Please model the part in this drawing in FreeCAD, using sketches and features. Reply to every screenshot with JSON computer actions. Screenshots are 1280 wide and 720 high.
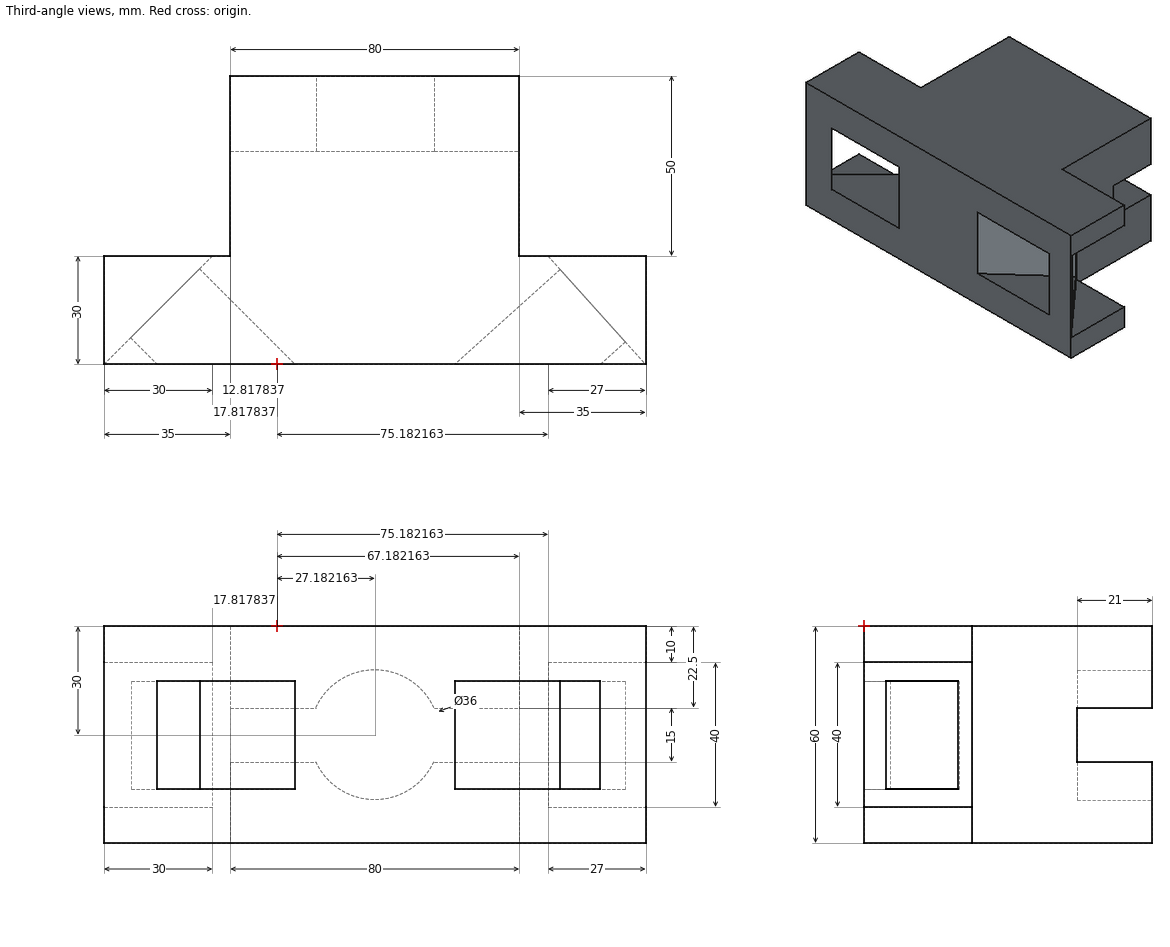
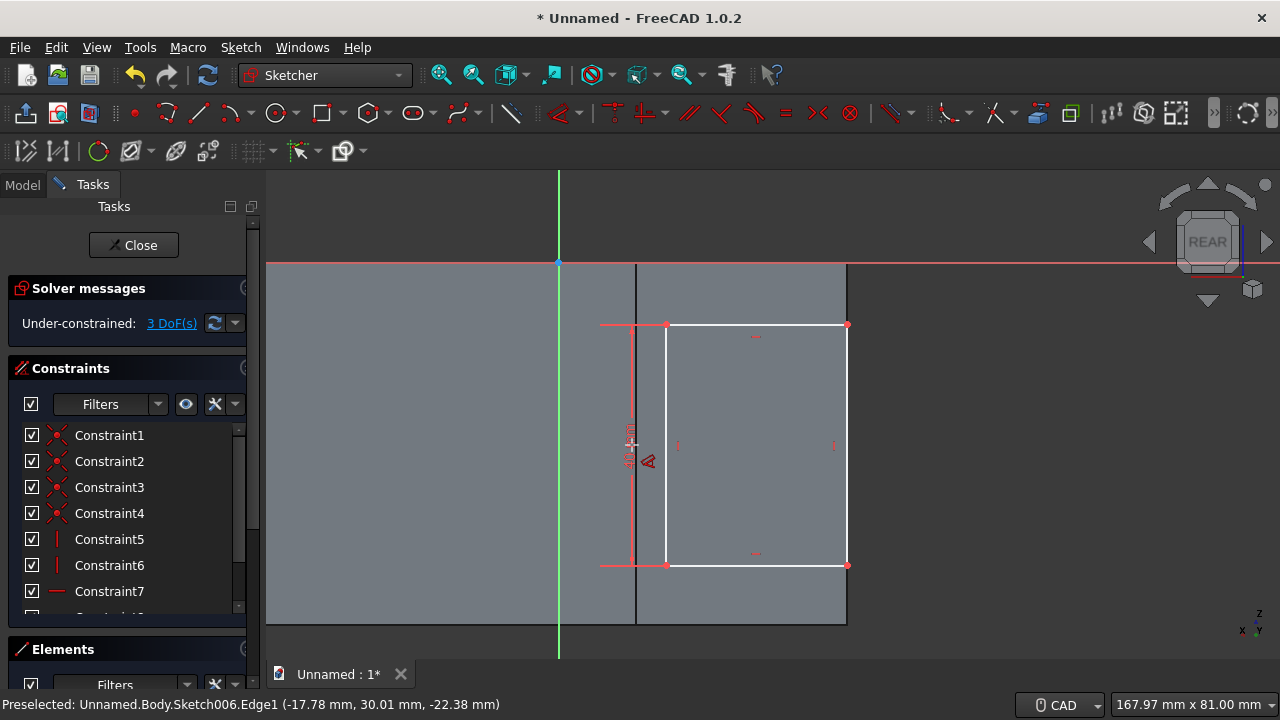
{"action": "left_click", "coordinate": [720, 566]}
{"action": "left_click", "coordinate": [757, 600]}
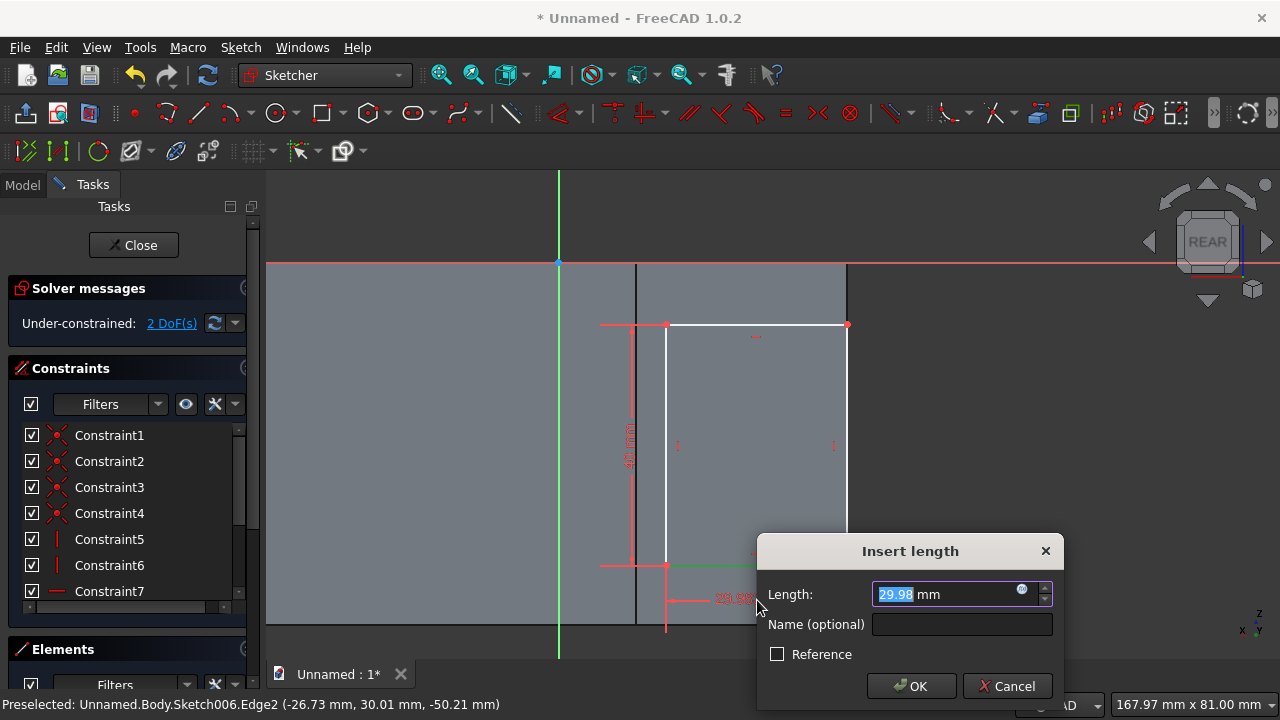
{"action": "type", "text": "30"}
{"action": "key", "text": "Return"}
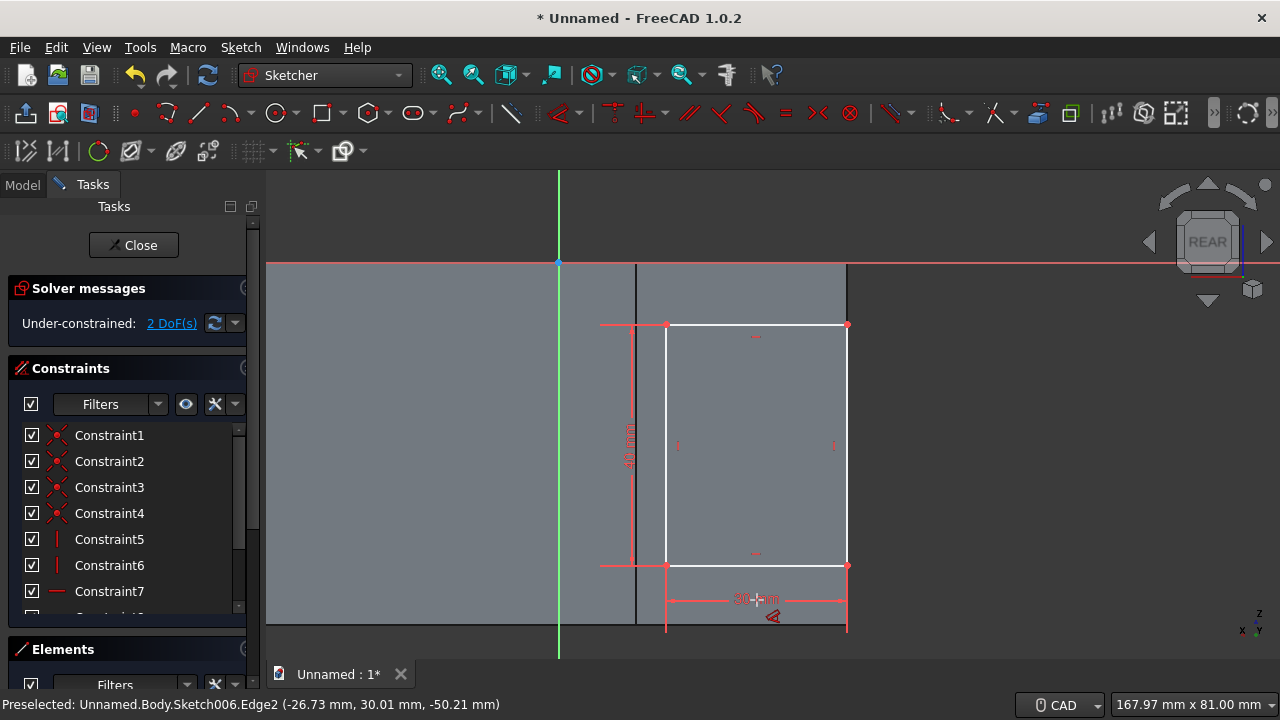
{"action": "left_click", "coordinate": [666, 325]}
{"action": "left_click", "coordinate": [525, 294]}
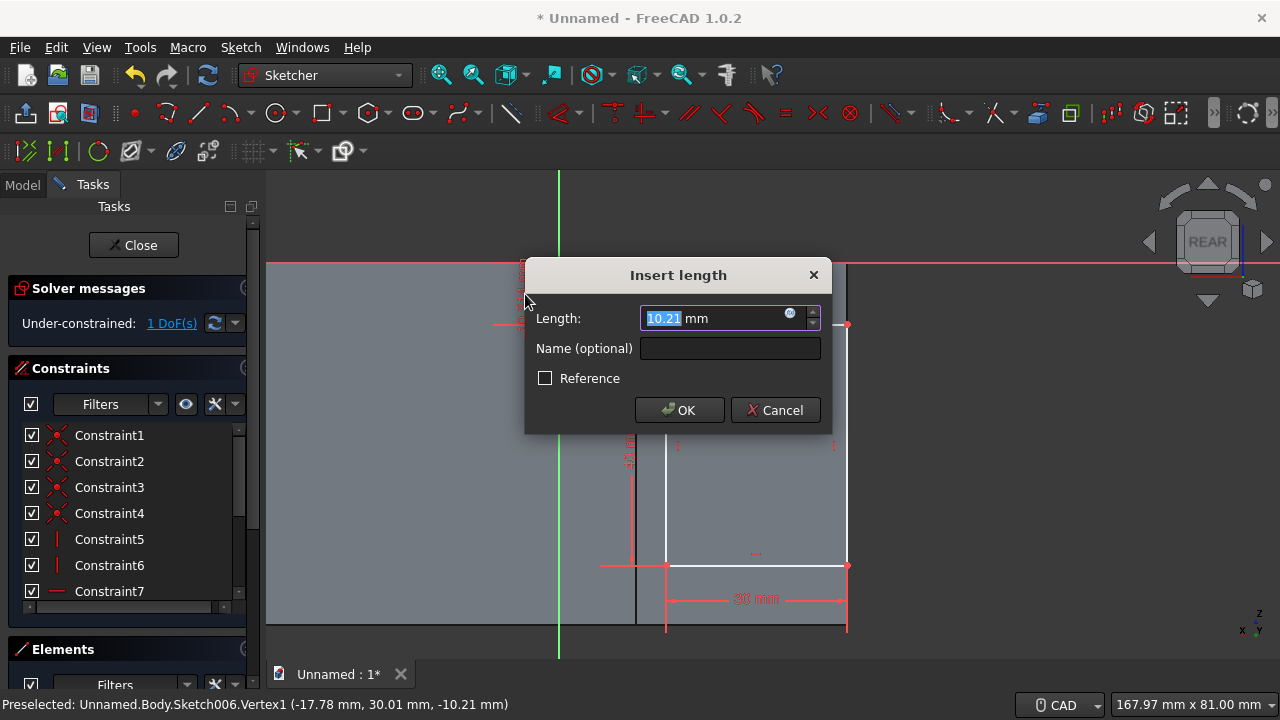
{"action": "type", "text": "10"}
{"action": "key", "text": "Return"}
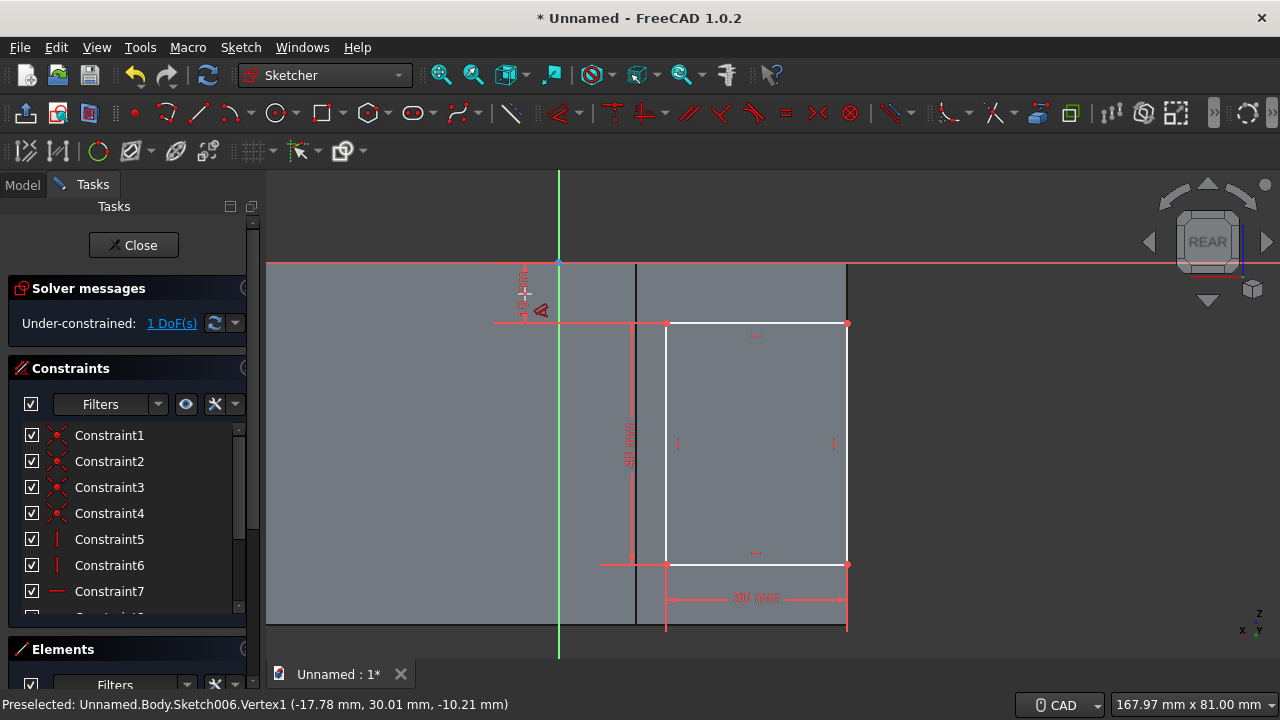
{"action": "left_click", "coordinate": [666, 323]}
{"action": "left_click", "coordinate": [612, 229]}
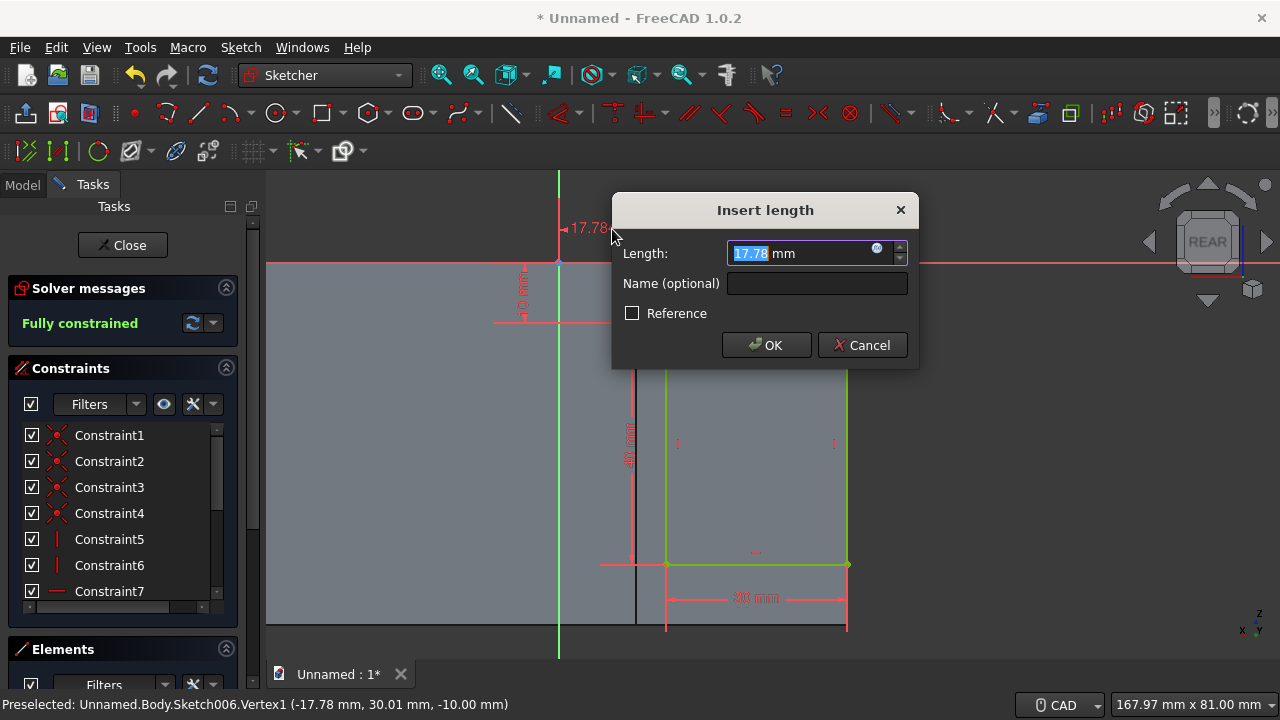
{"action": "type", "text": "17.817837"}
{"action": "key", "text": "Return"}
{"action": "key", "text": "Escape"}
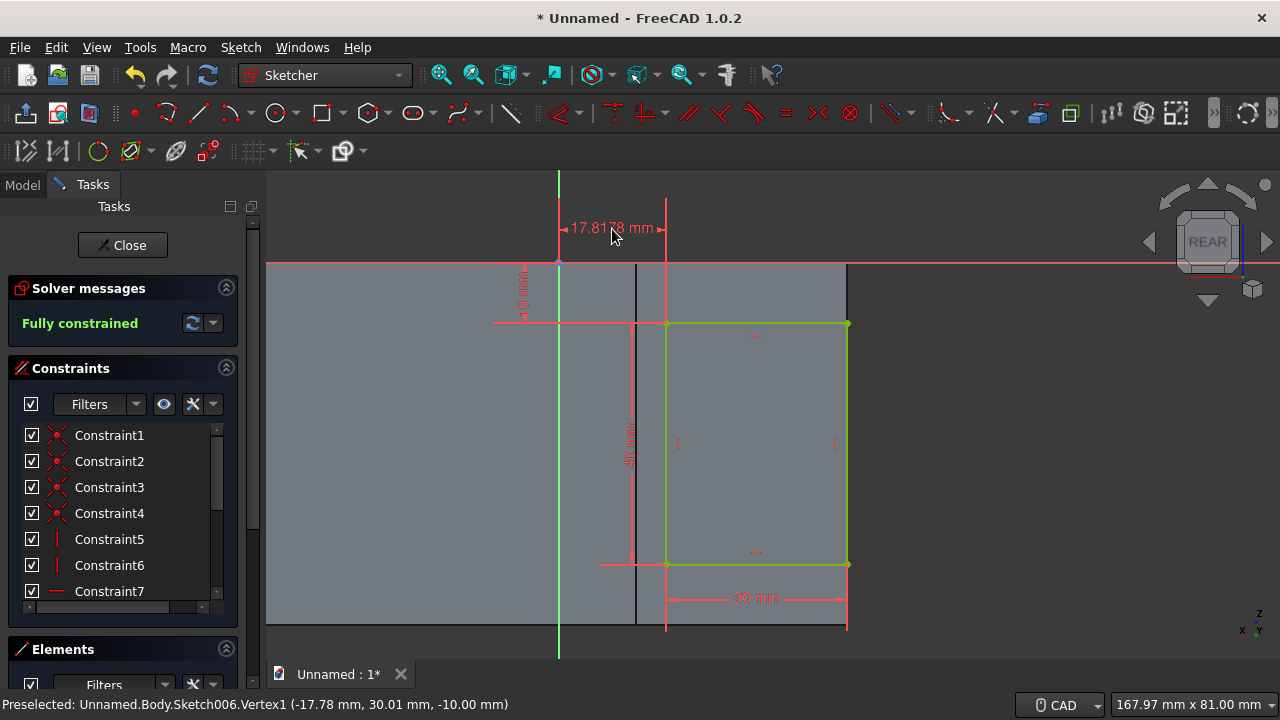
{"action": "left_click", "coordinate": [123, 245]}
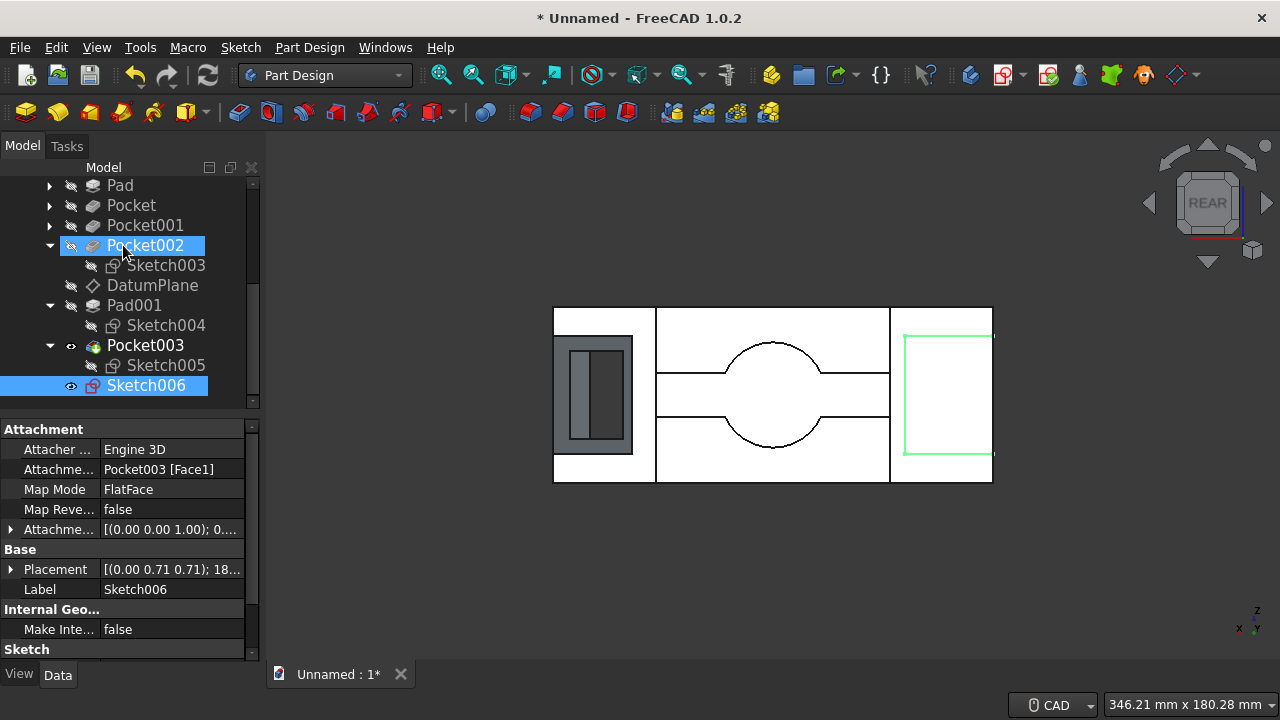
{"action": "left_click", "coordinate": [240, 112]}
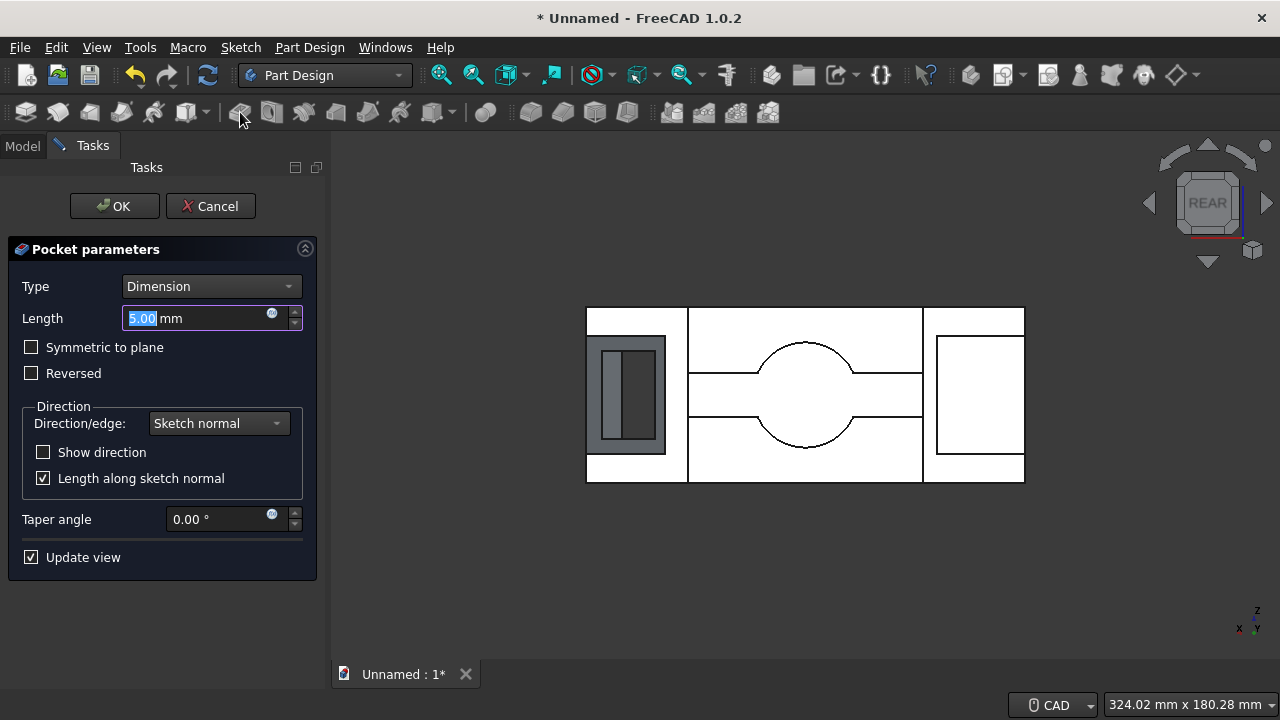
{"action": "type", "text": "40"}
{"action": "key", "text": "Tab"}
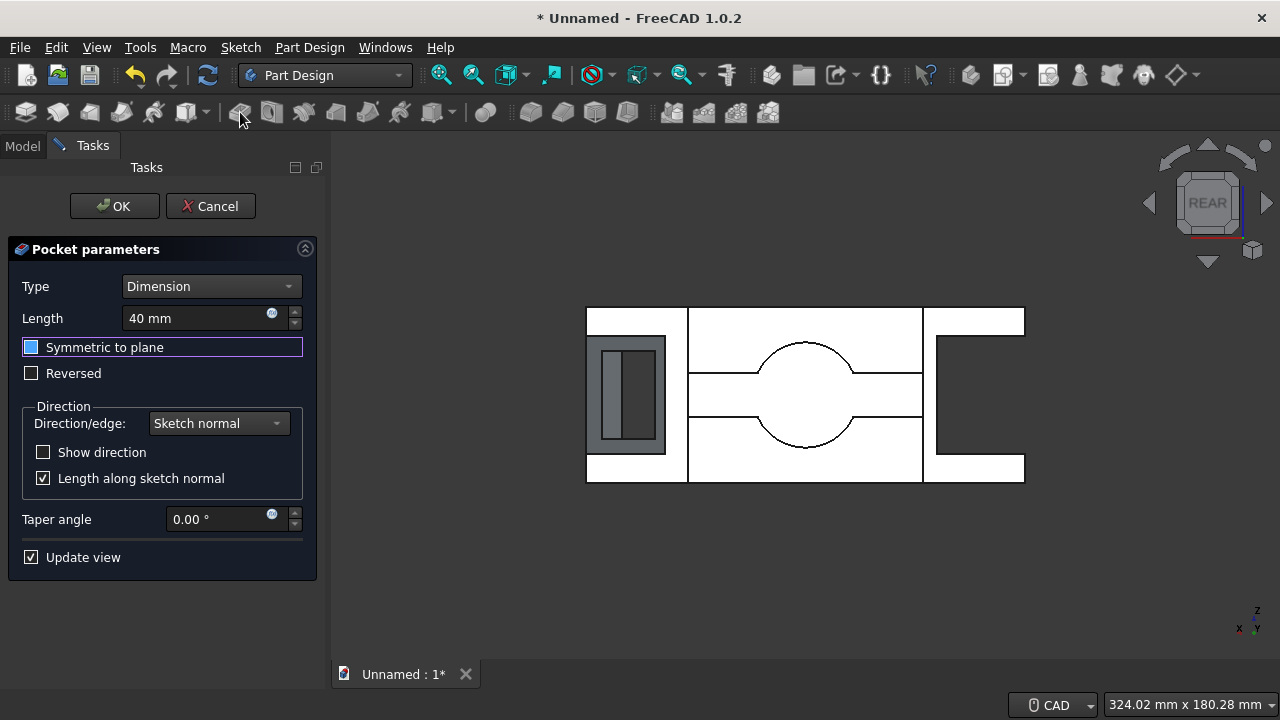
{"action": "left_click", "coordinate": [115, 206]}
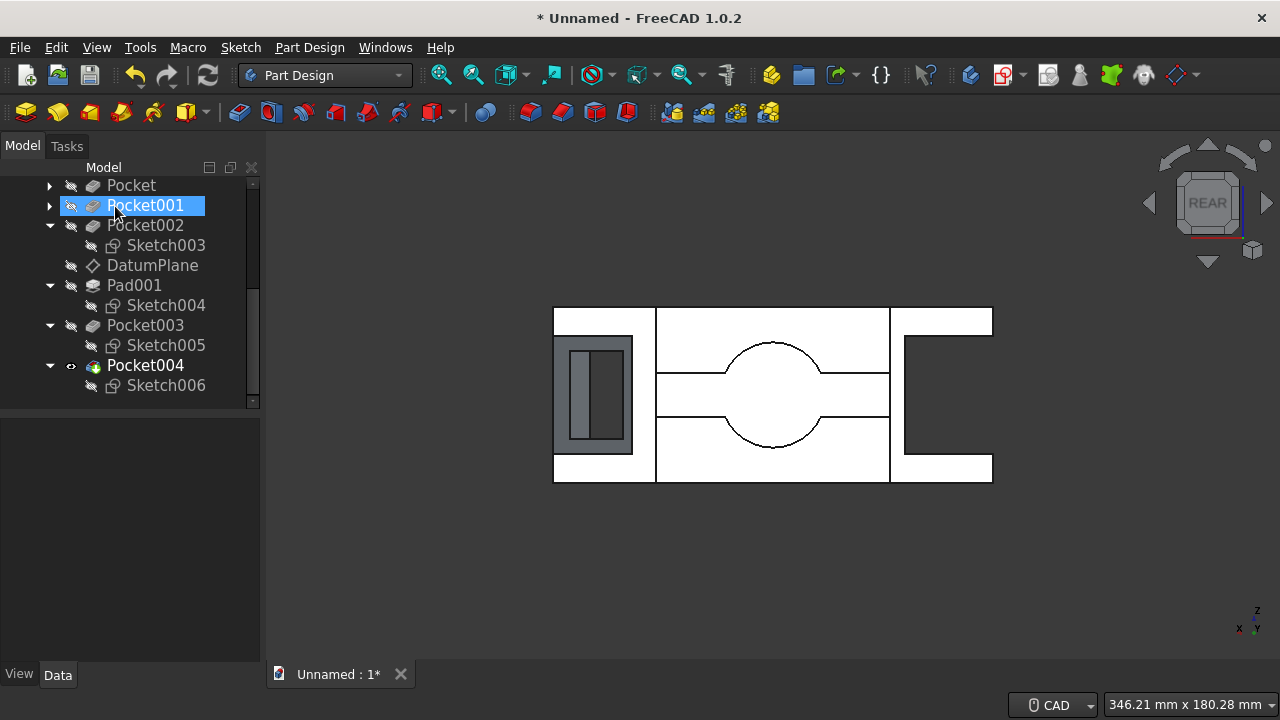
{"action": "left_click", "coordinate": [442, 76]}